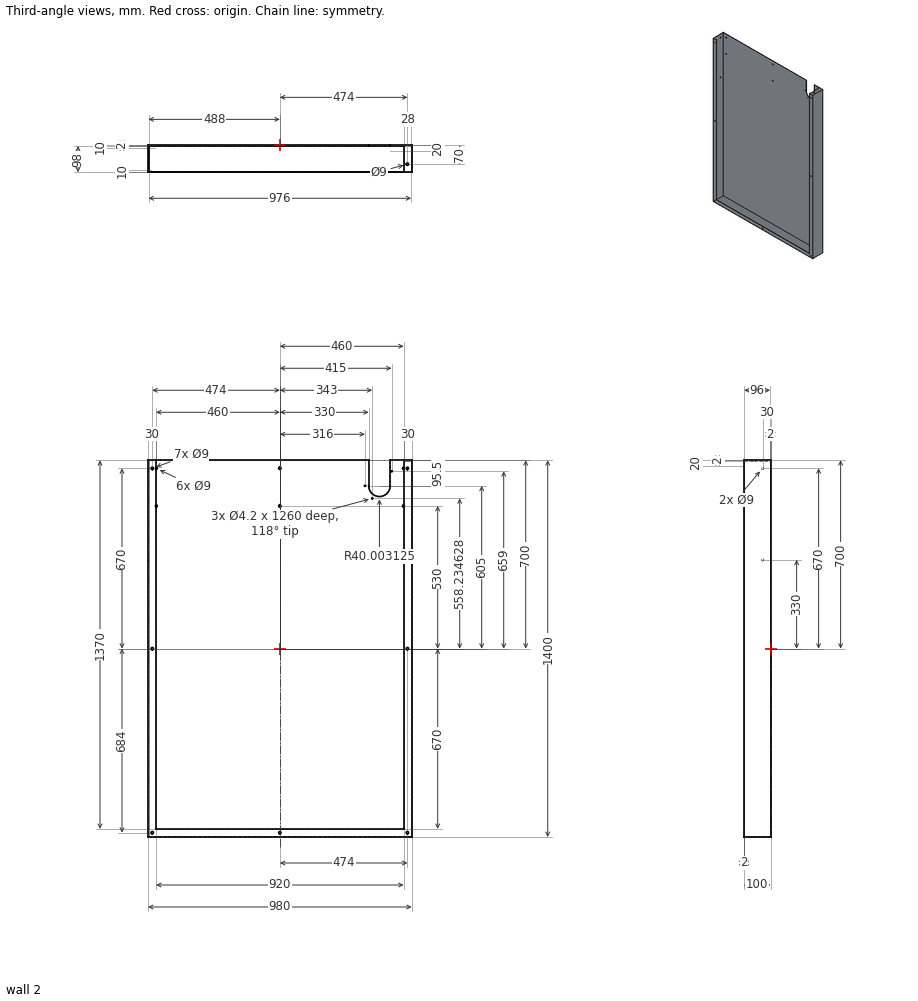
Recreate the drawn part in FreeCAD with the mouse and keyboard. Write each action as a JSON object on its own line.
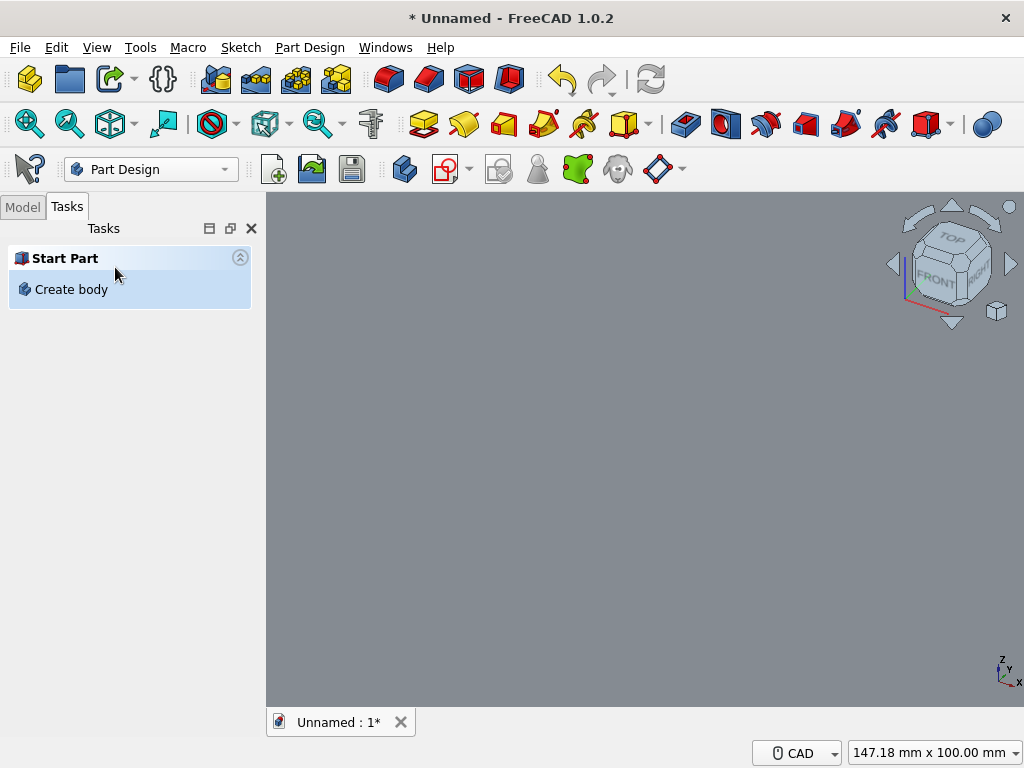
{"action": "left_click", "coordinate": [30, 124]}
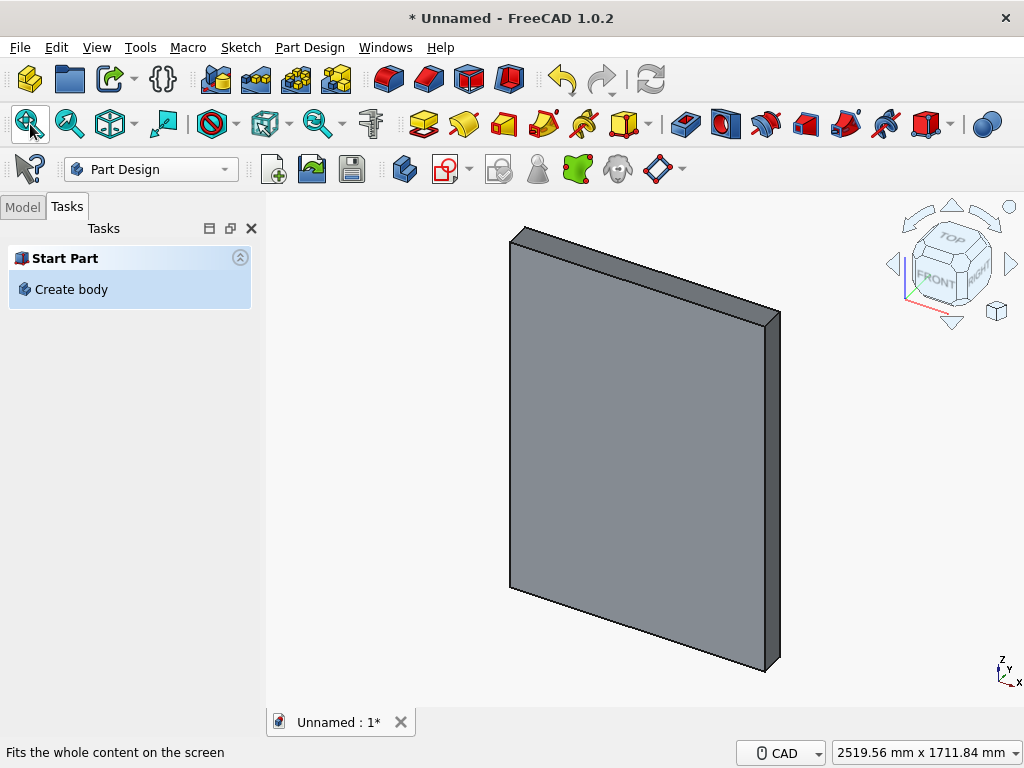
{"action": "left_click", "coordinate": [637, 407]}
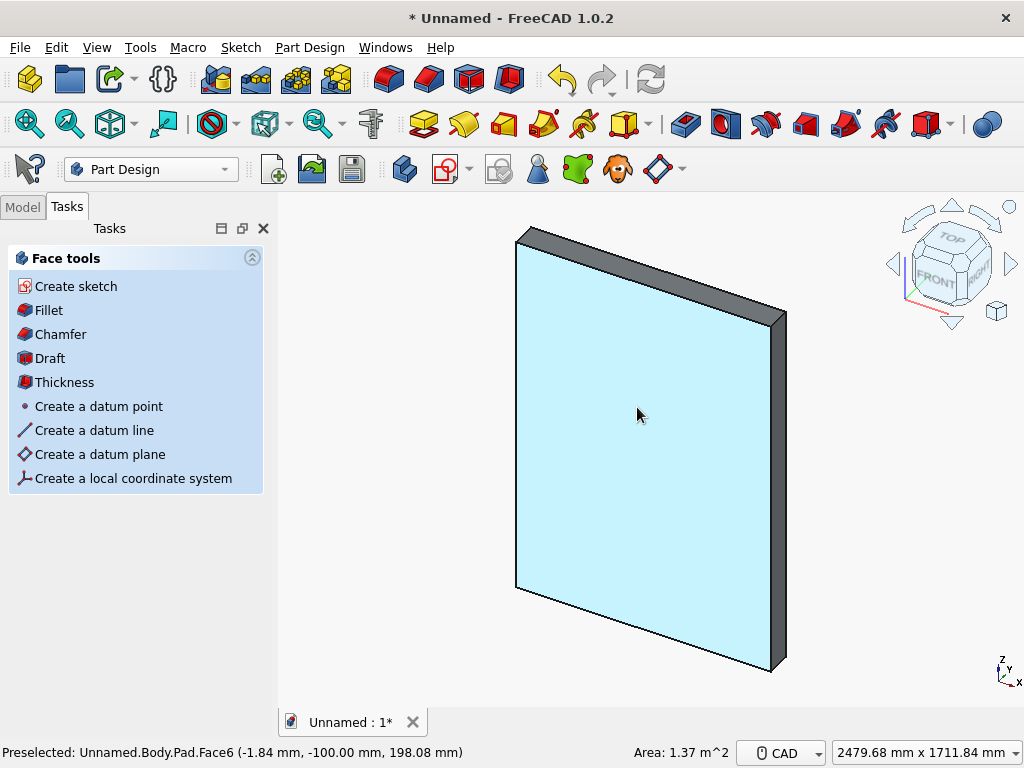
{"action": "left_click", "coordinate": [510, 80]}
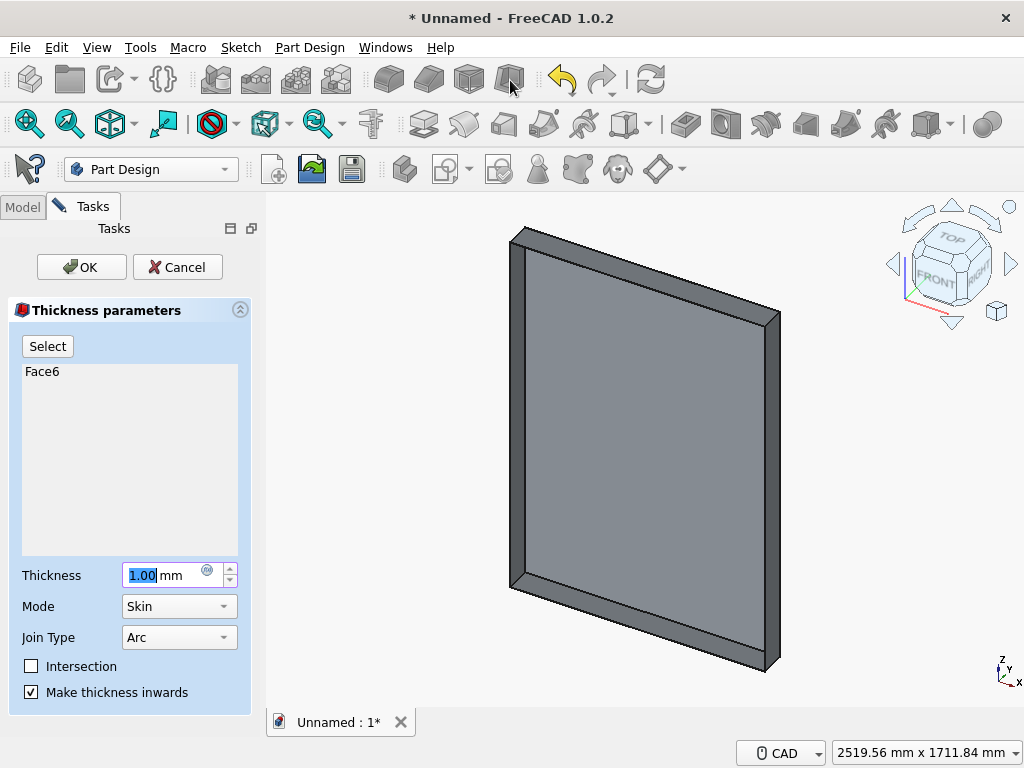
{"action": "type", "text": "2"}
{"action": "key", "text": "Tab"}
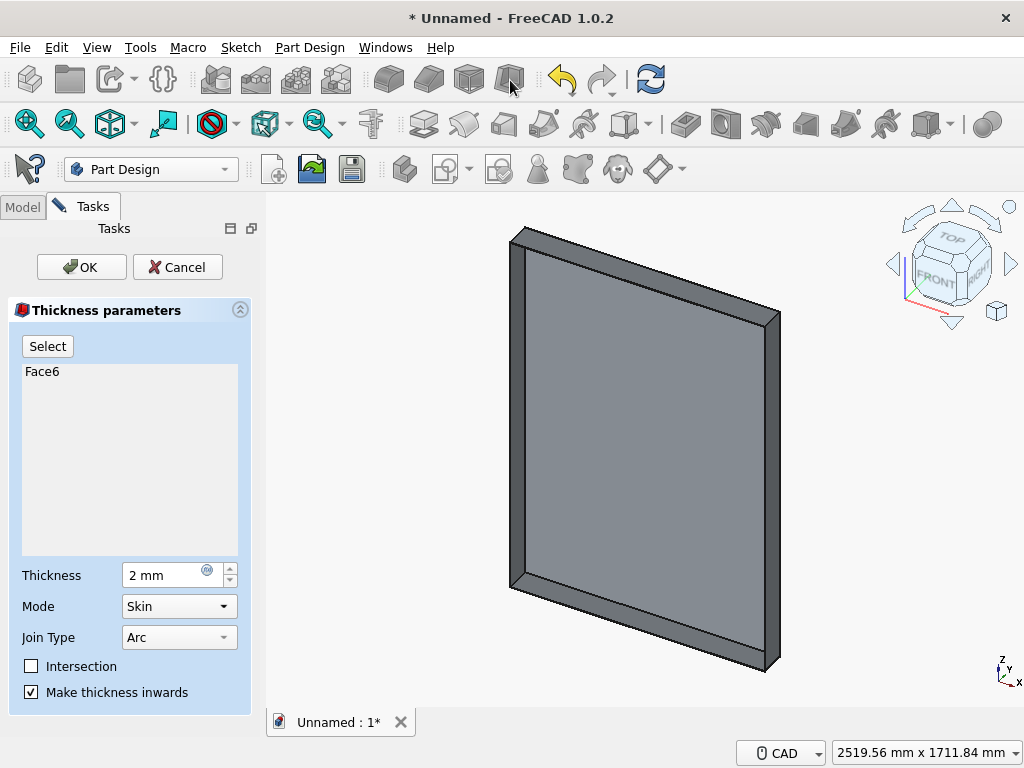
{"action": "left_click", "coordinate": [180, 638]}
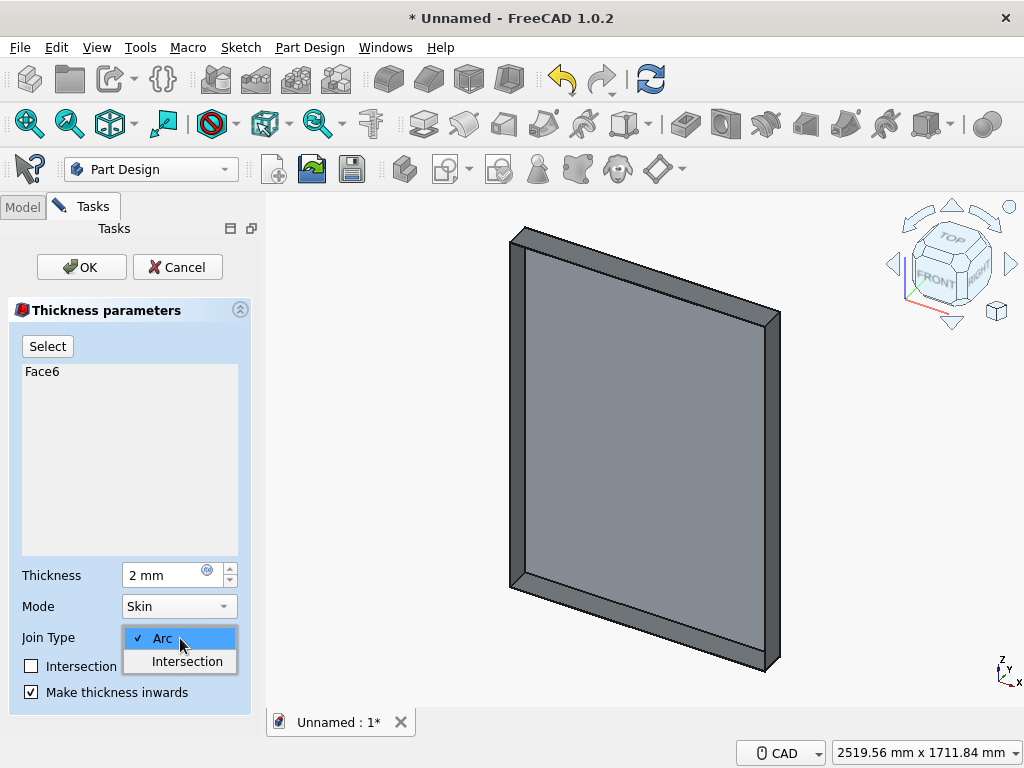
{"action": "left_click", "coordinate": [179, 662]}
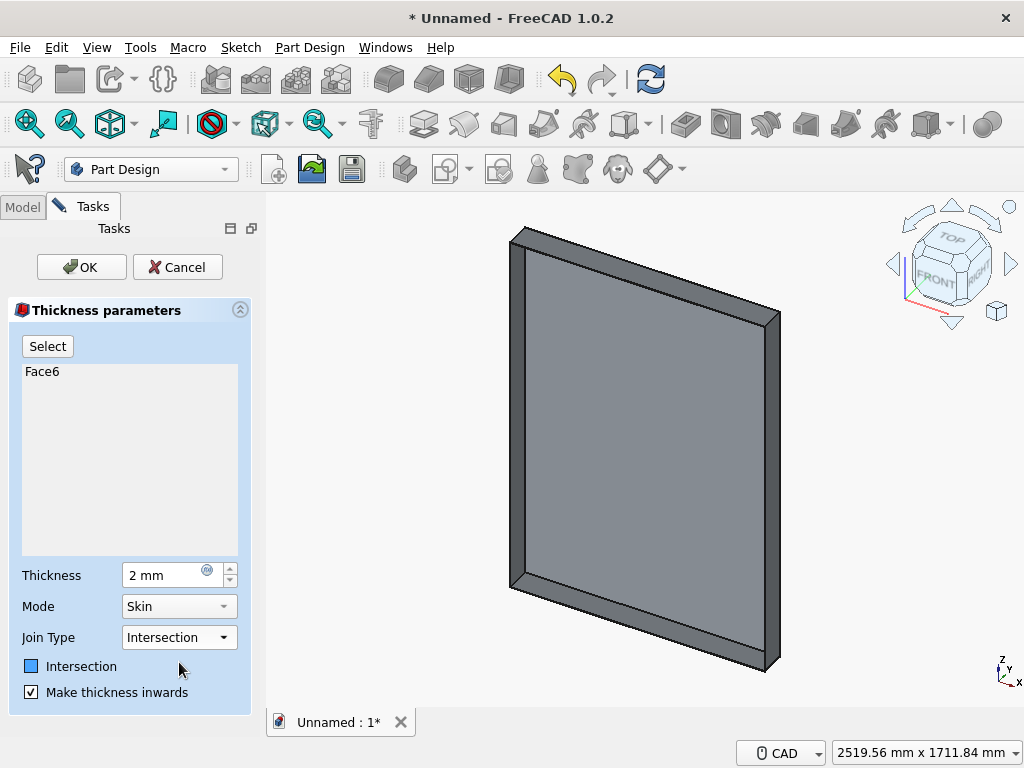
{"action": "left_click", "coordinate": [82, 267]}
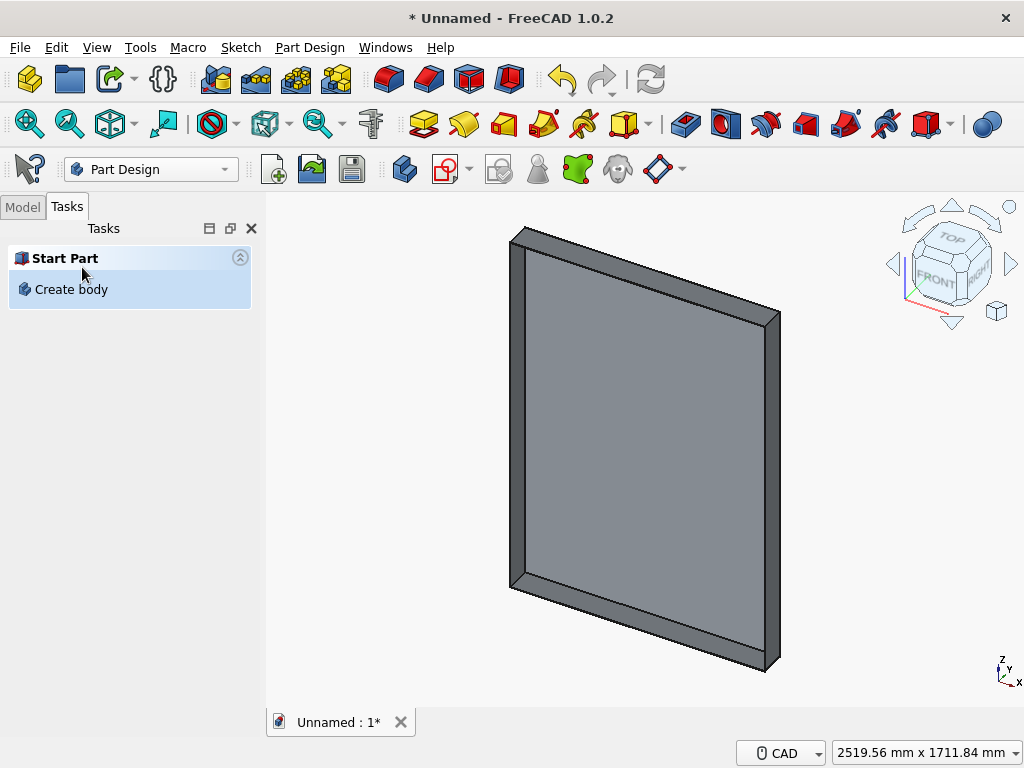
{"action": "key", "text": "4"}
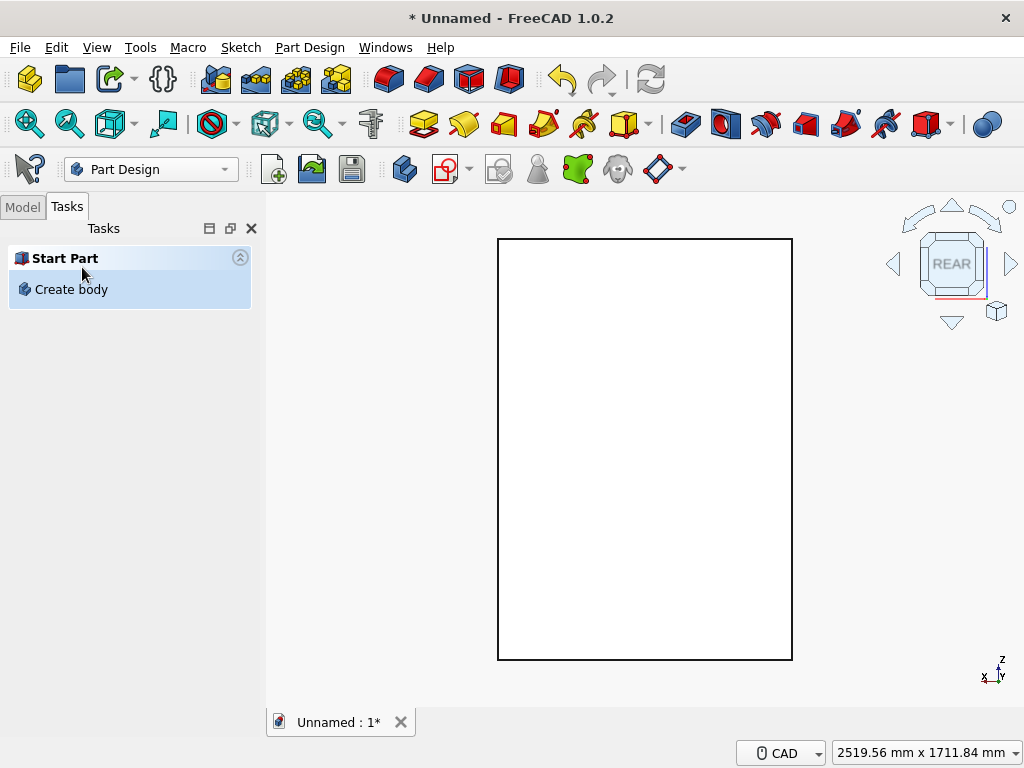
{"action": "left_click", "coordinate": [645, 388]}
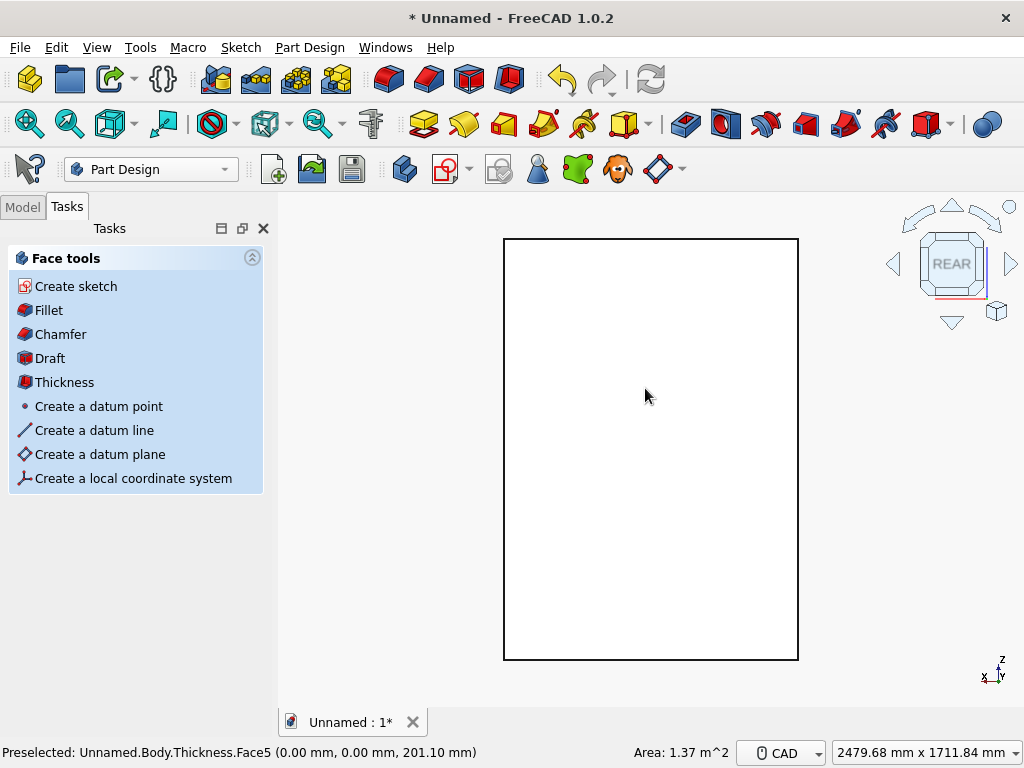
{"action": "left_click", "coordinate": [446, 170]}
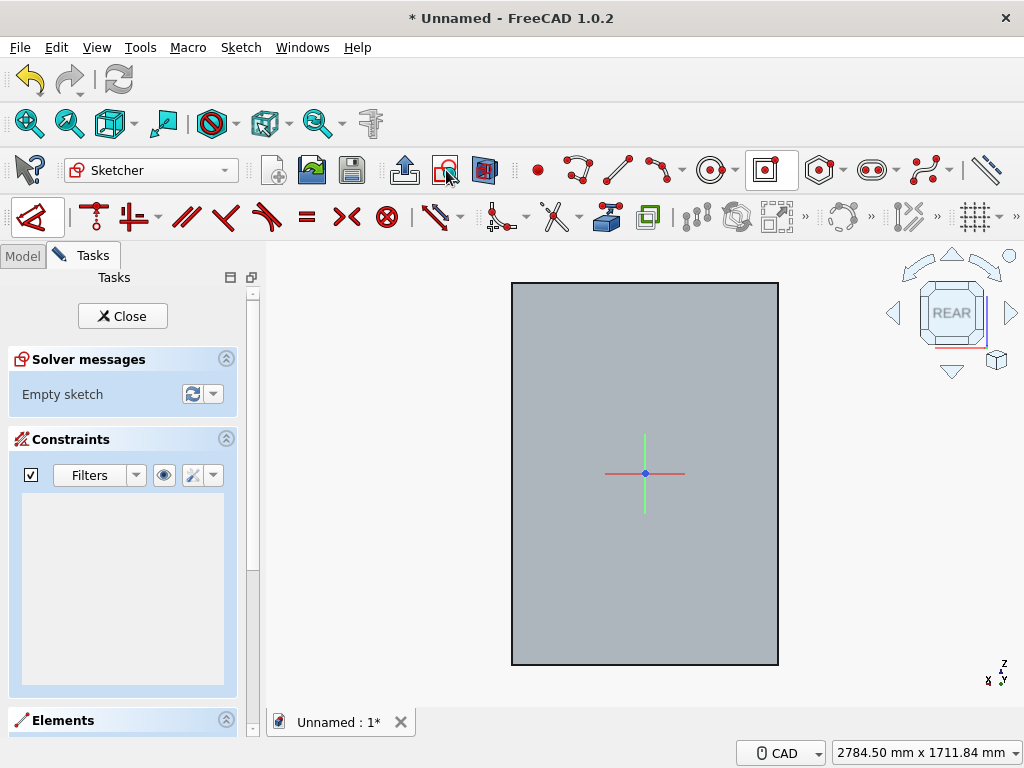
{"action": "scroll", "coordinate": [539, 275], "scroll_direction": "up", "scroll_amount": 10}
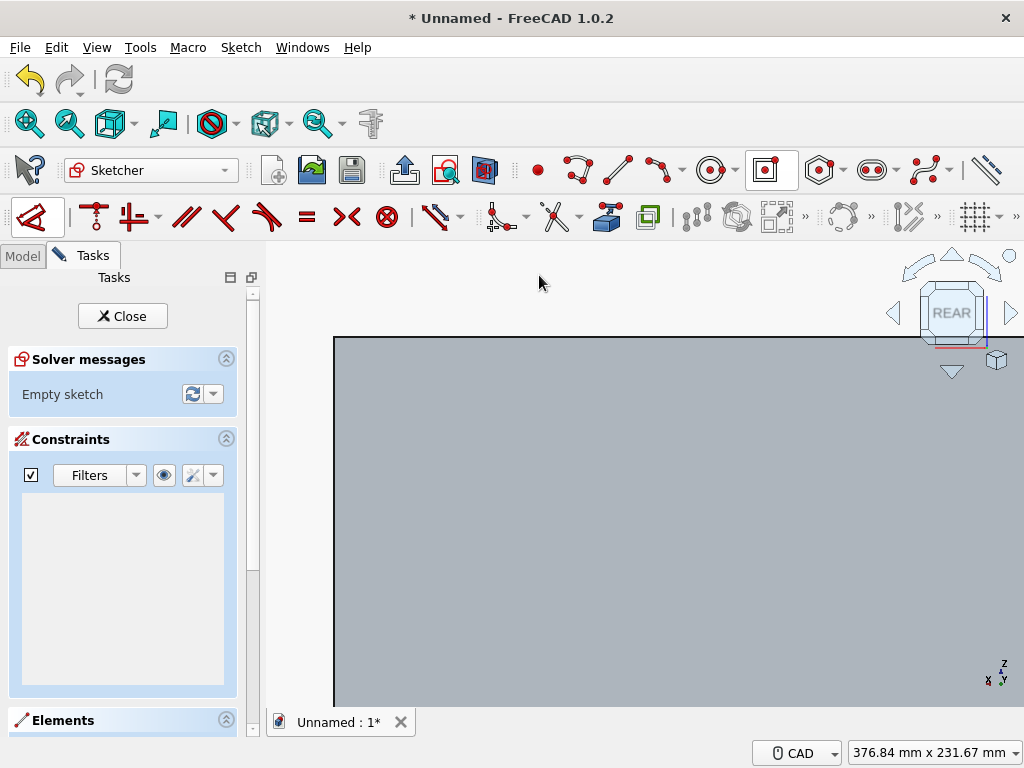
{"action": "left_click", "coordinate": [578, 170]}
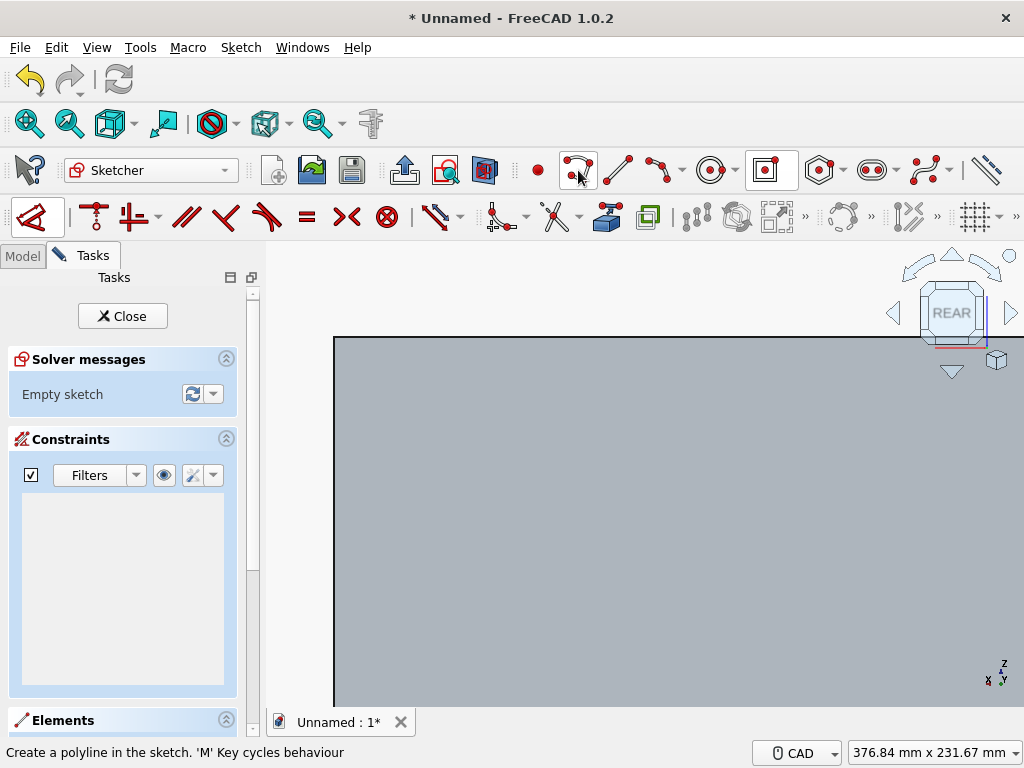
{"action": "left_click", "coordinate": [656, 529]}
{"action": "left_click", "coordinate": [656, 337]}
{"action": "left_click", "coordinate": [495, 337]}
{"action": "left_click", "coordinate": [495, 529]}
{"action": "right_click", "coordinate": [495, 529]}